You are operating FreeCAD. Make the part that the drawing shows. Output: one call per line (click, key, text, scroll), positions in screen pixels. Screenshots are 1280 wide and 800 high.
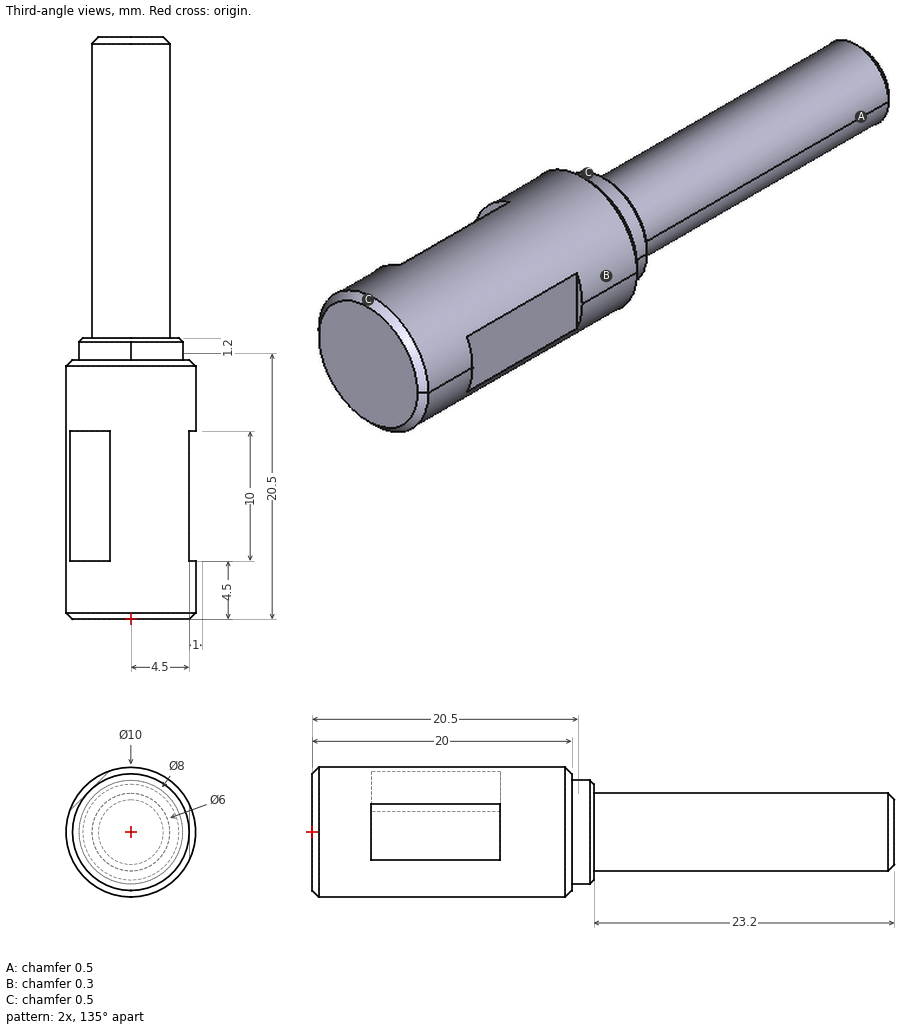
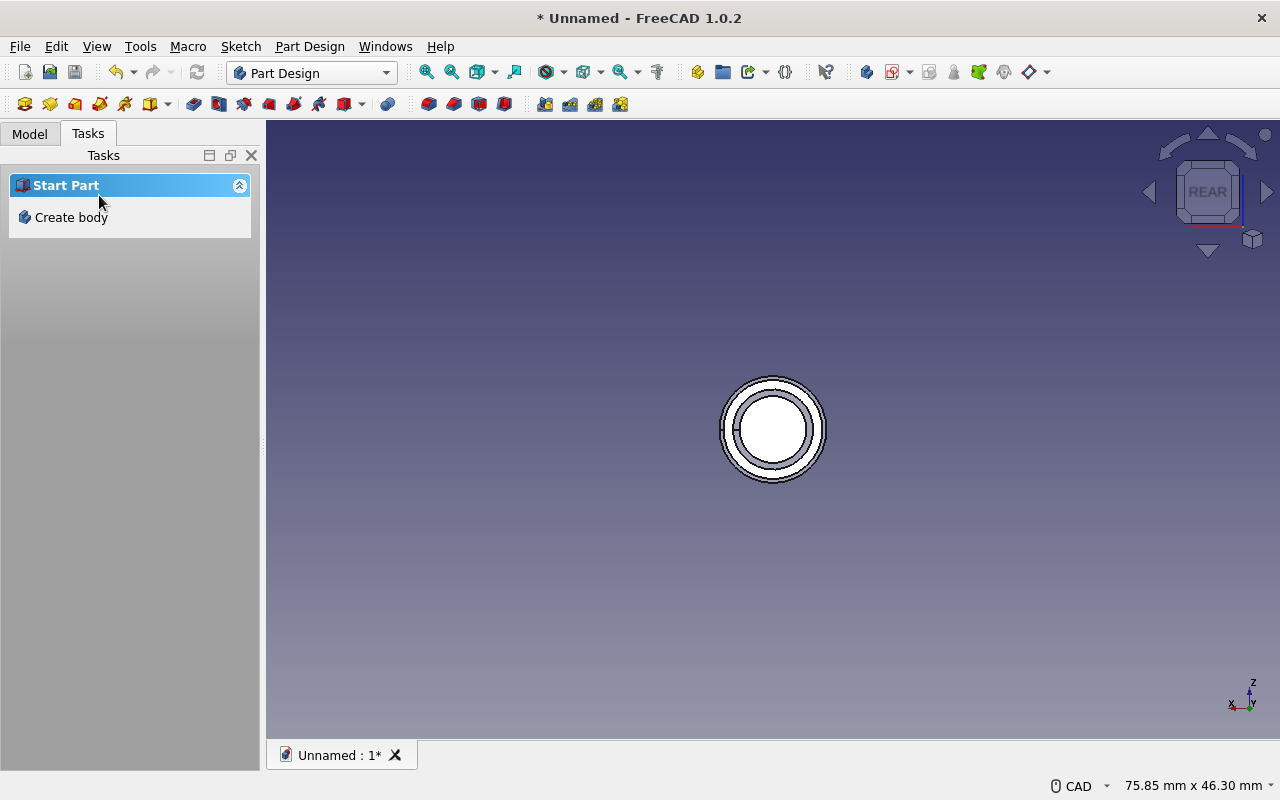
click(427, 72)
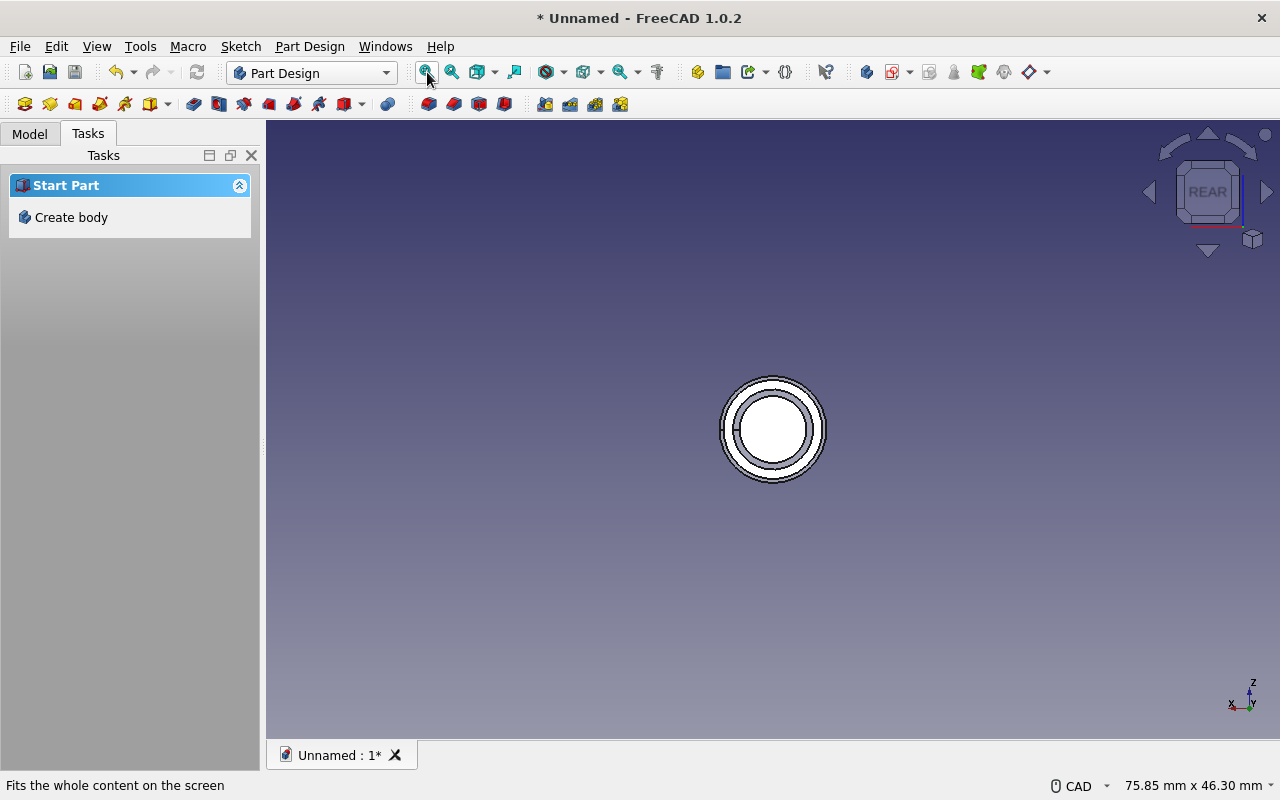
key(0)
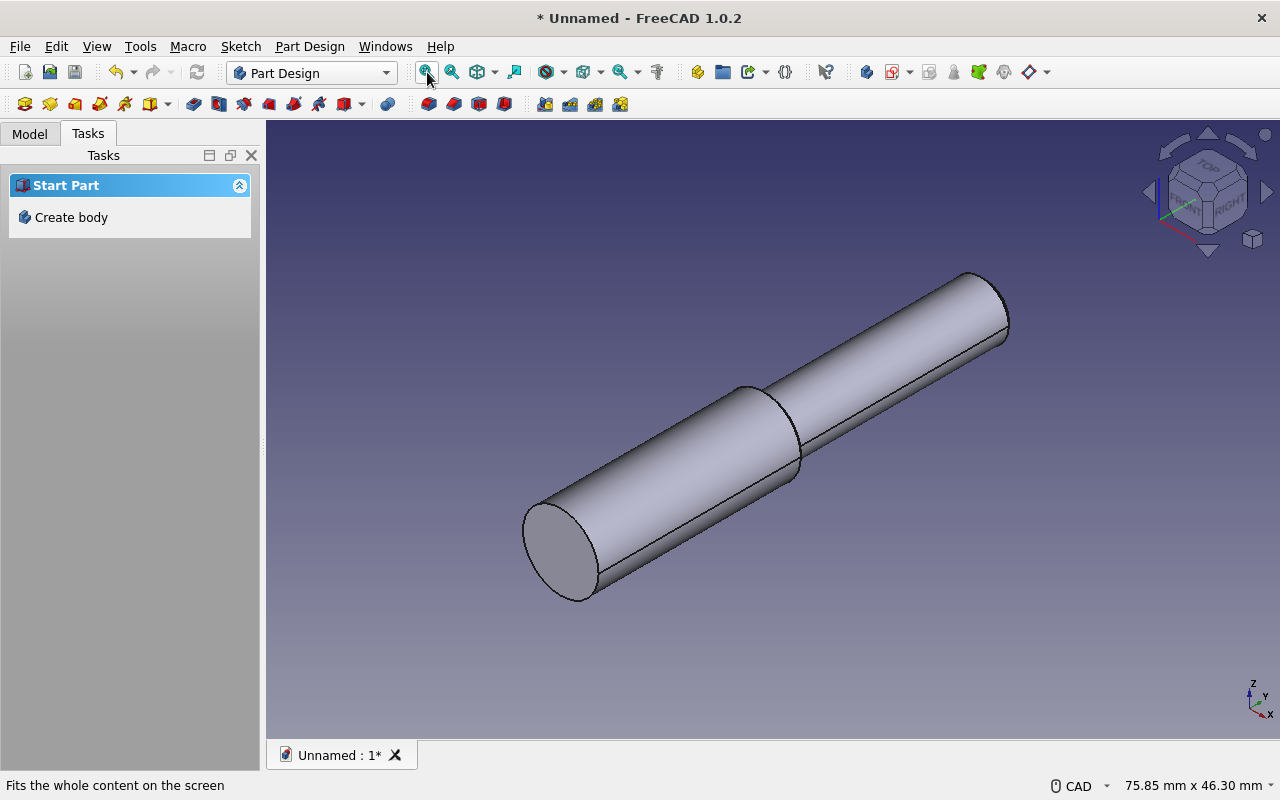
click(561, 551)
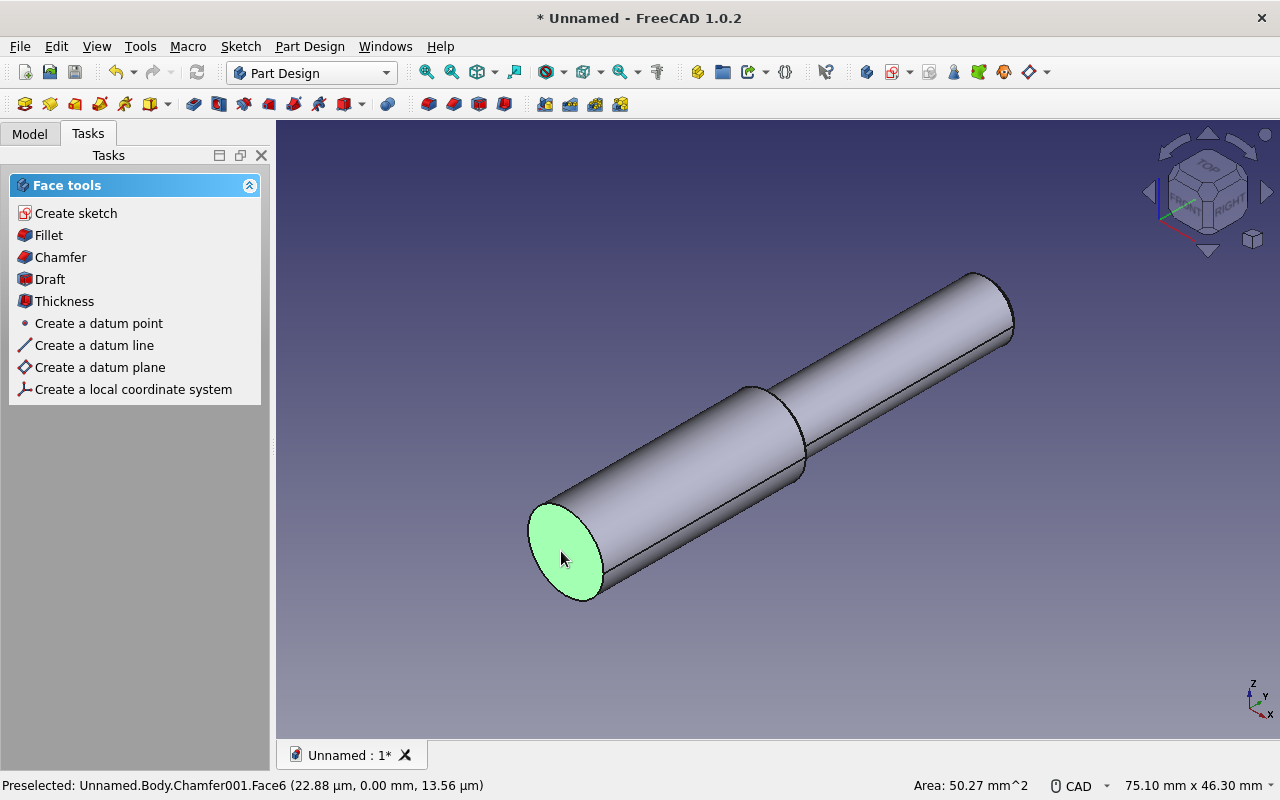
click(892, 72)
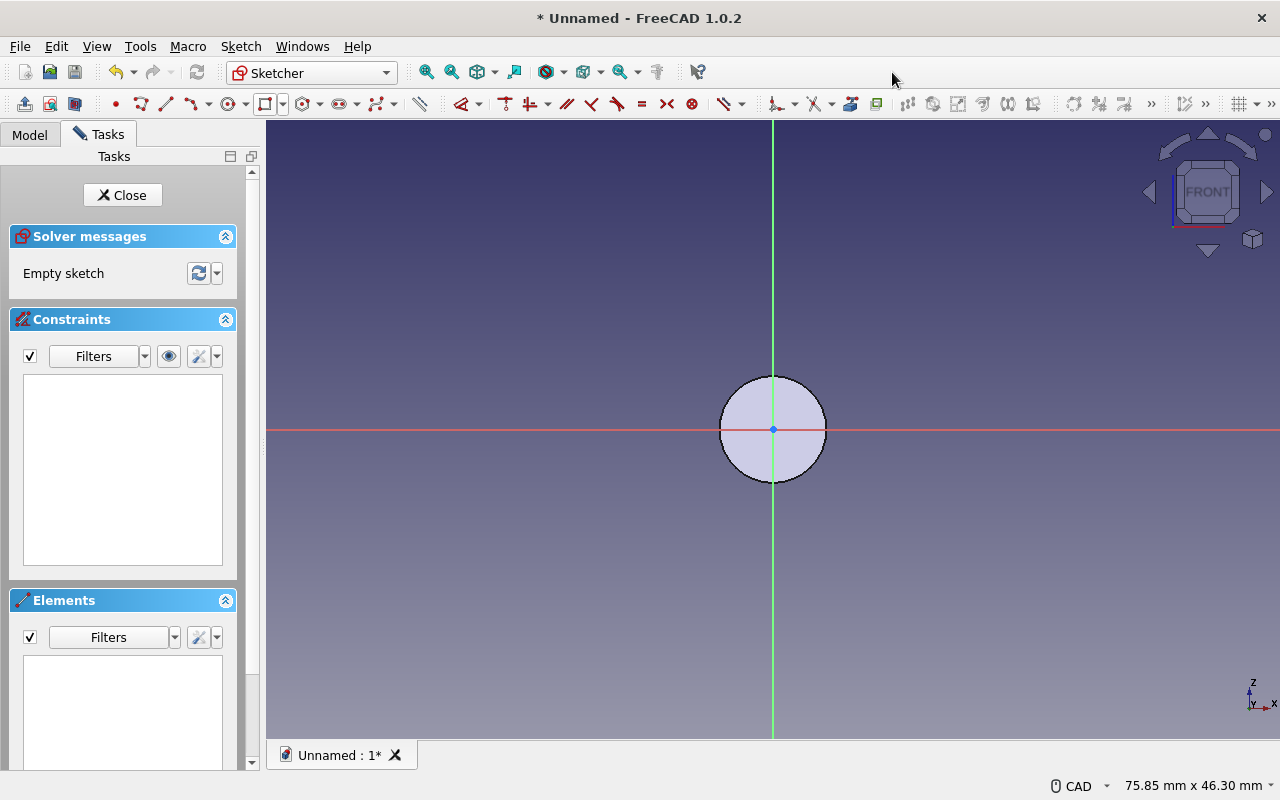
scroll(813, 430, up, 5)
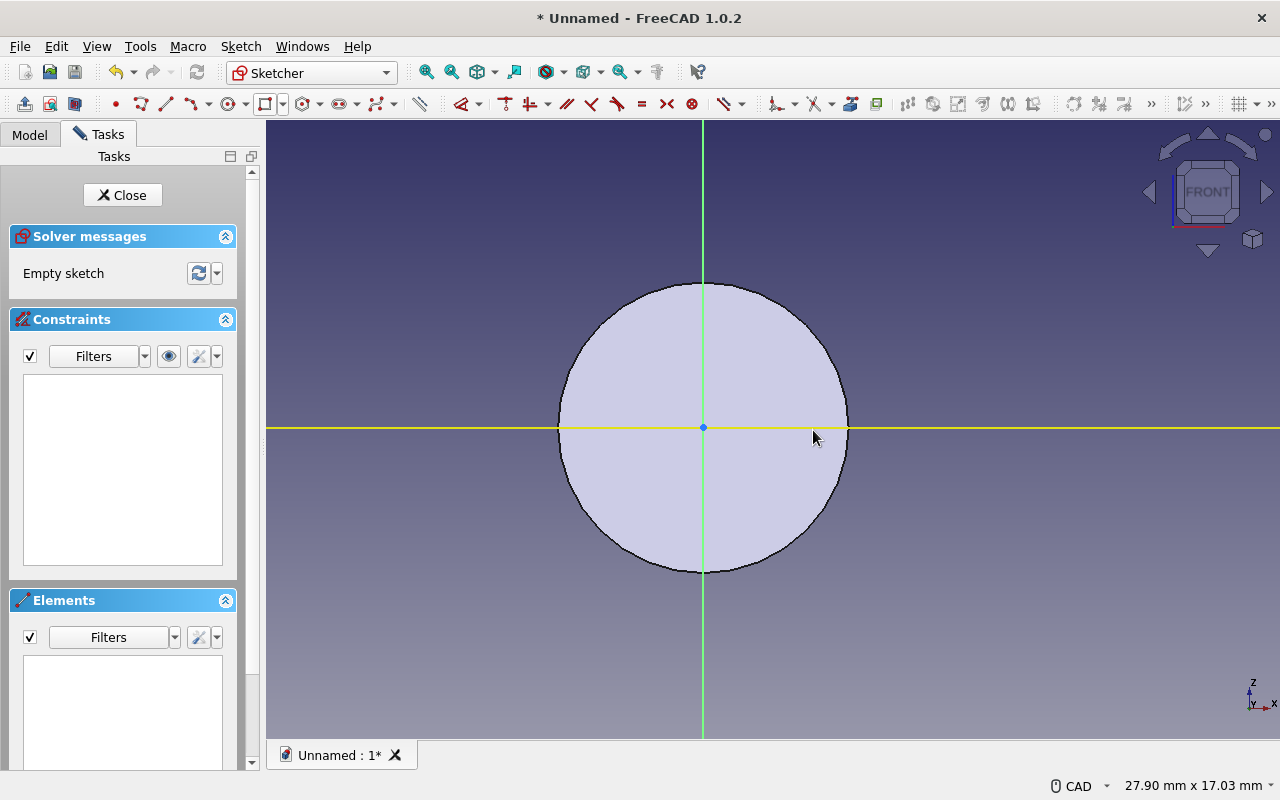
click(228, 104)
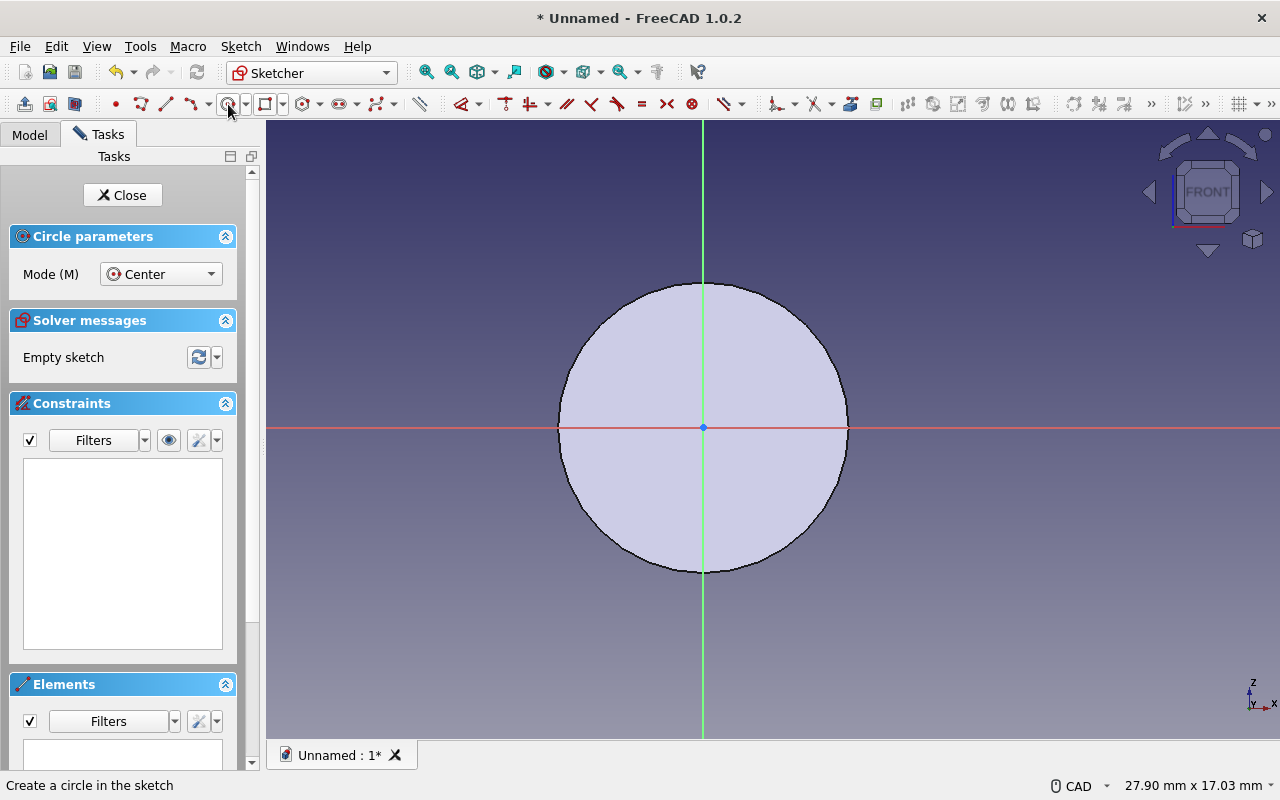
click(703, 428)
move(832, 299)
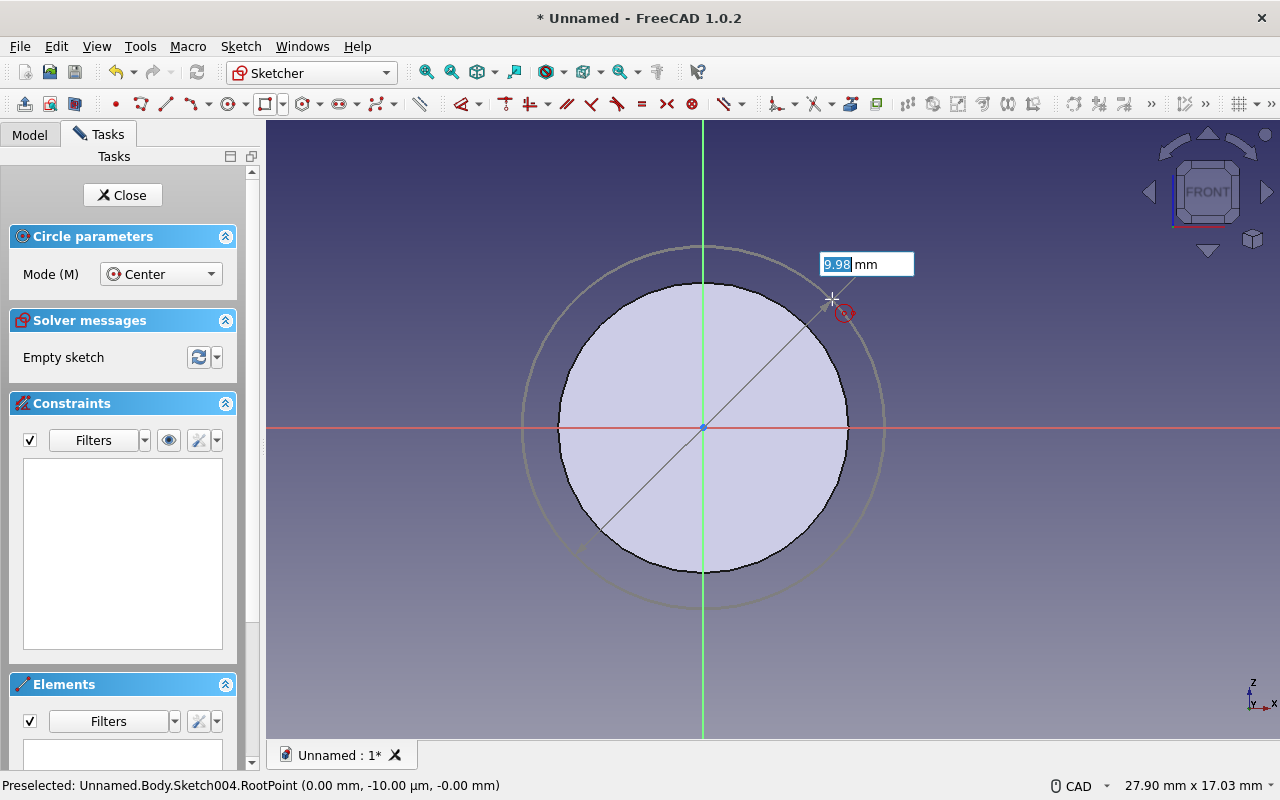
text(10)
key(Return)
key(Escape)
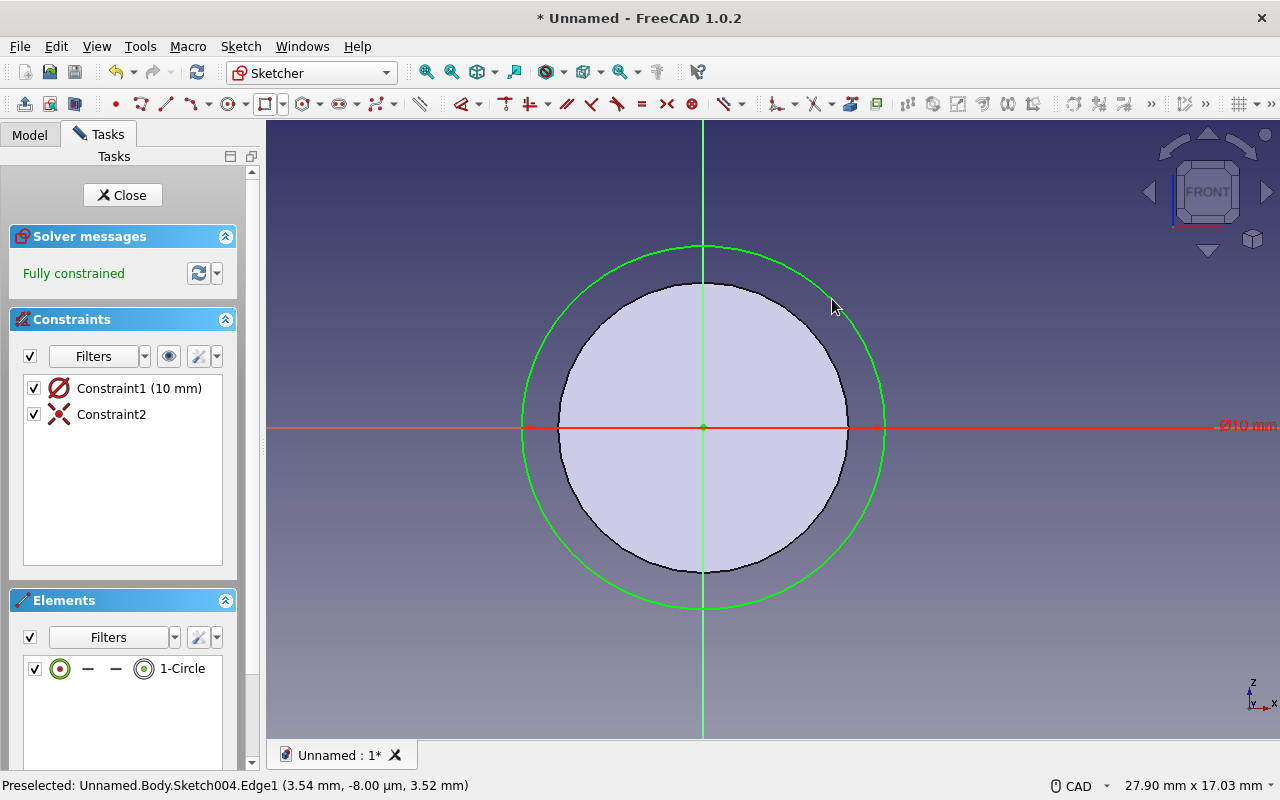
click(123, 195)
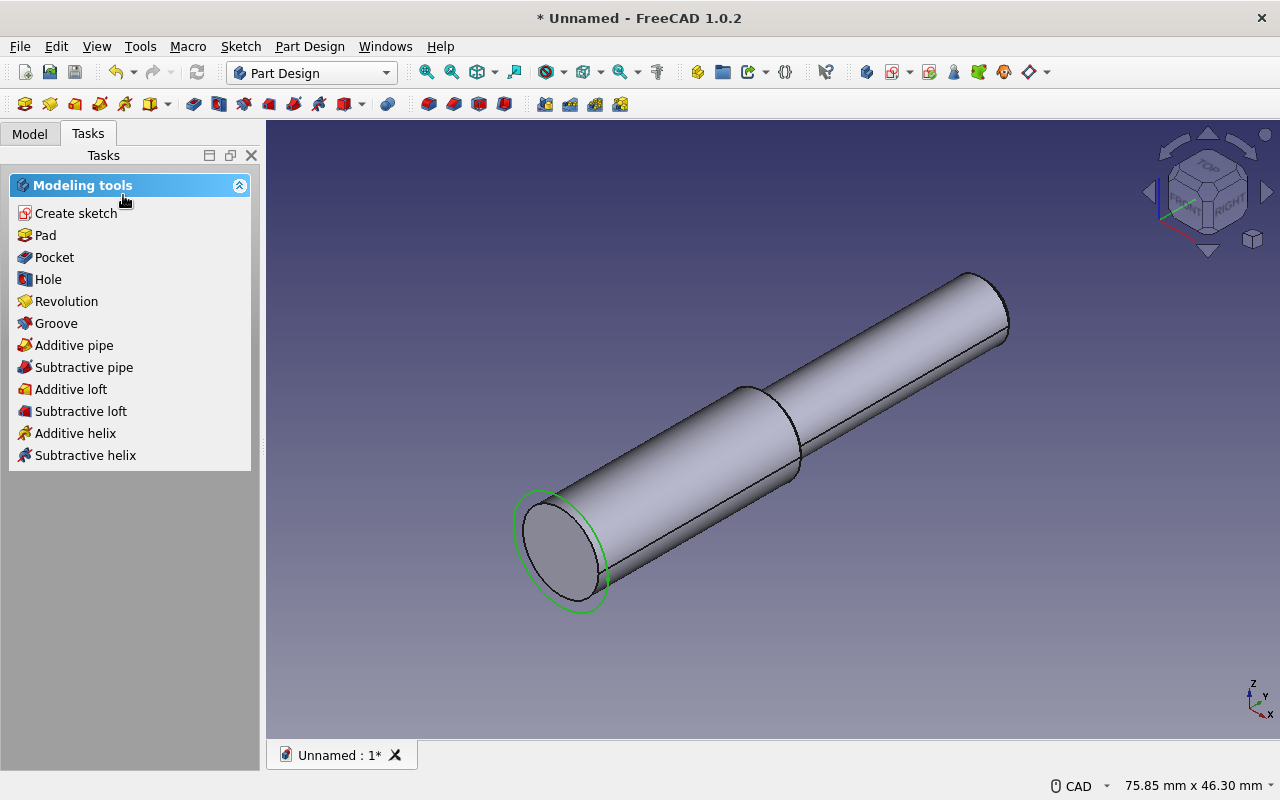
click(25, 104)